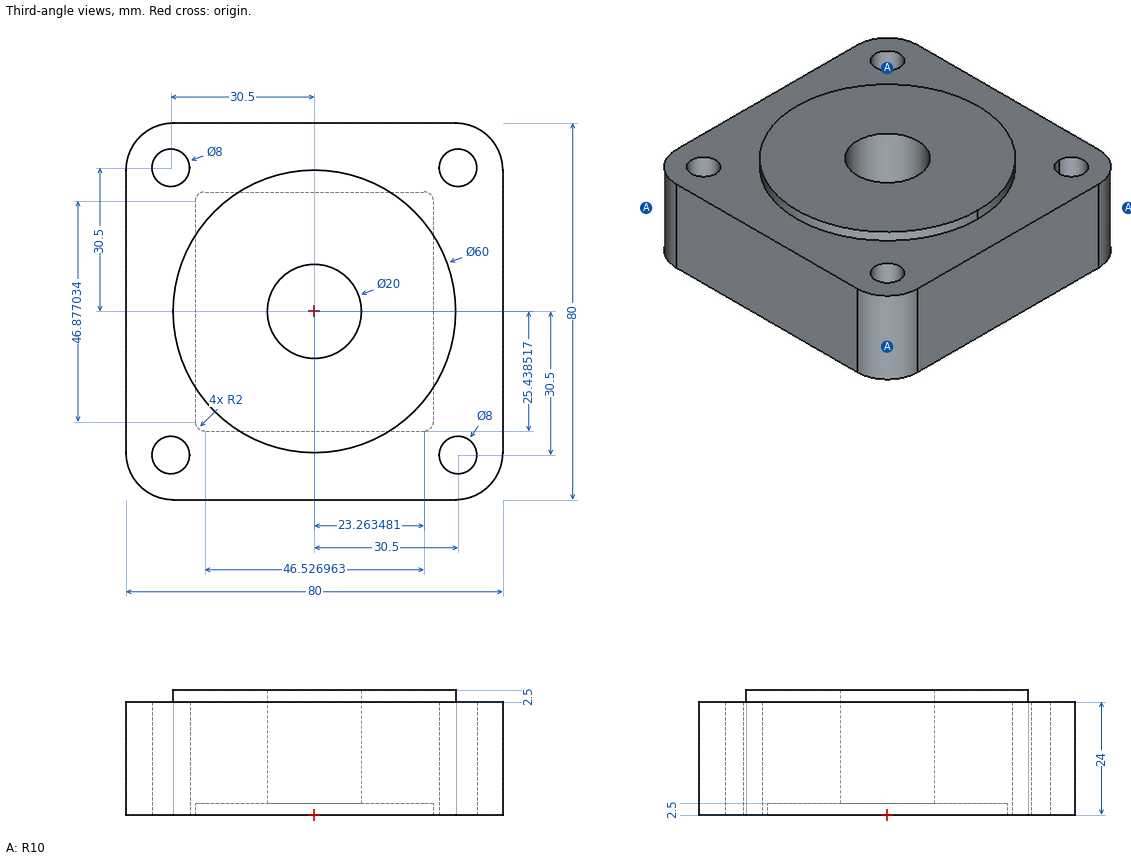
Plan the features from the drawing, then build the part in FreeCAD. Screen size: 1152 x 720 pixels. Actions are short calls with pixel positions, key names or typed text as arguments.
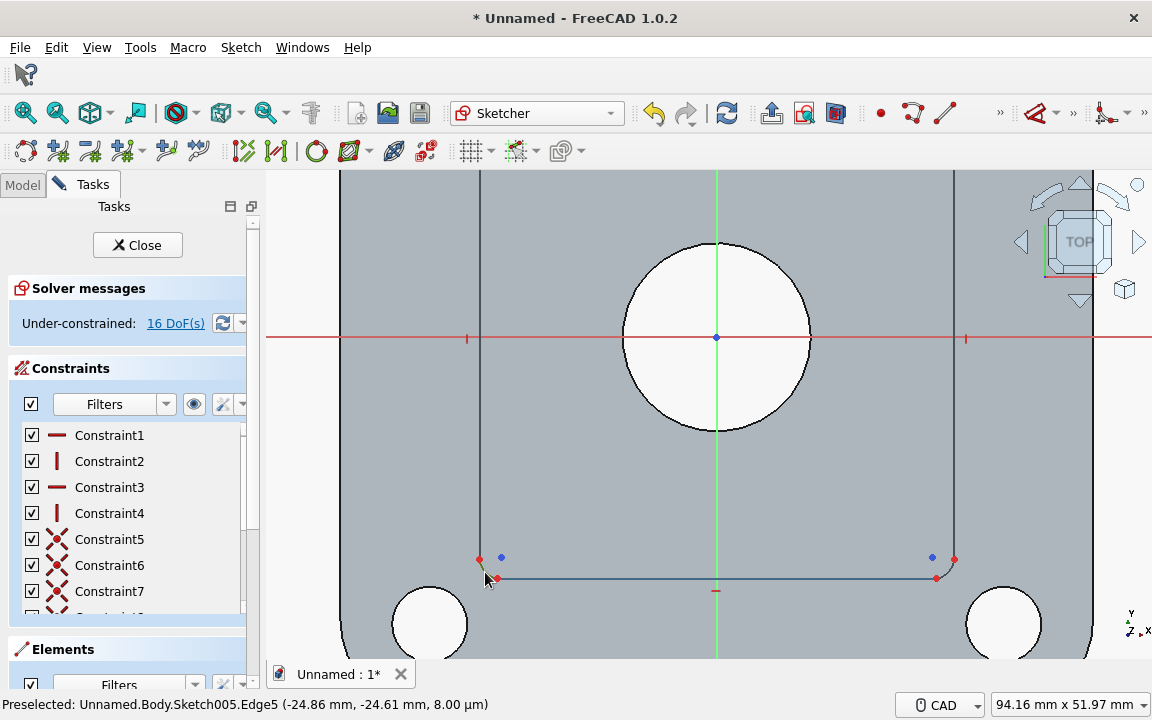
key(t)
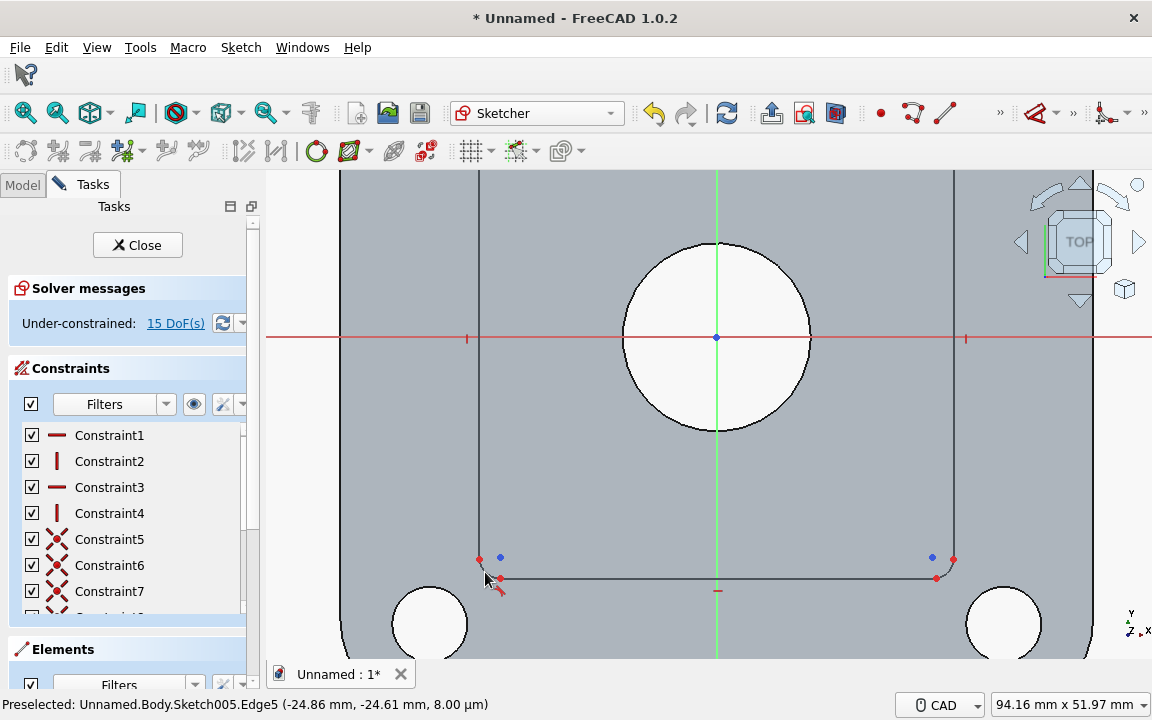
click(805, 579)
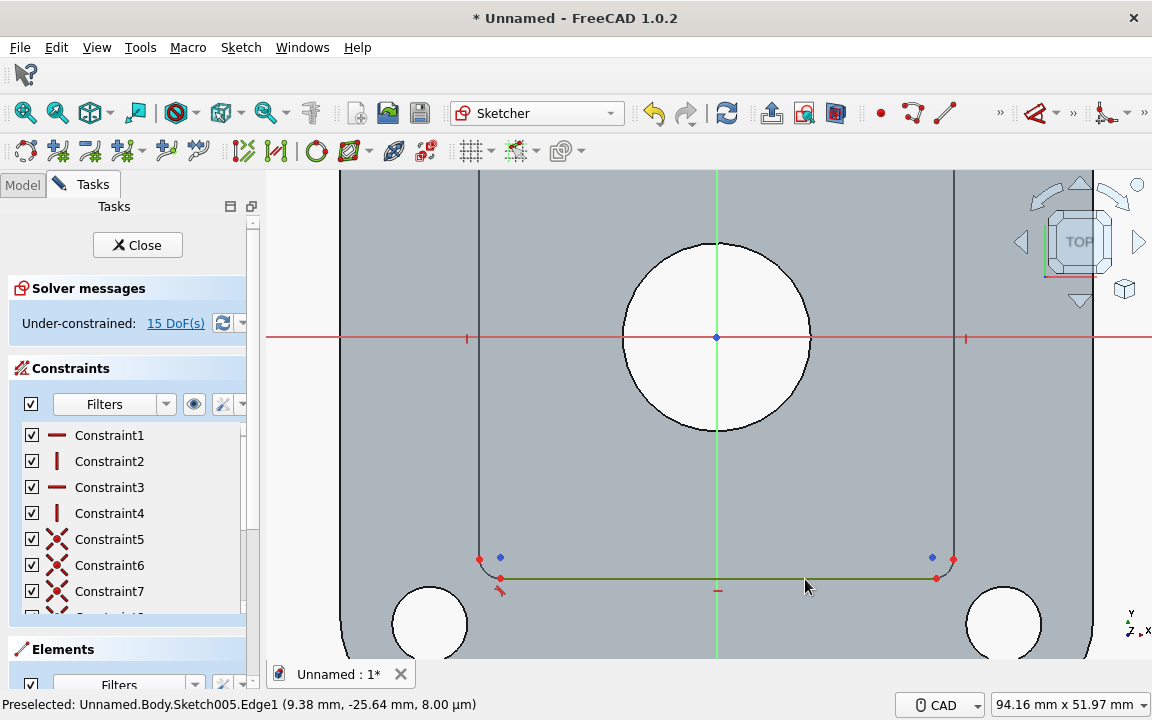
click(948, 572)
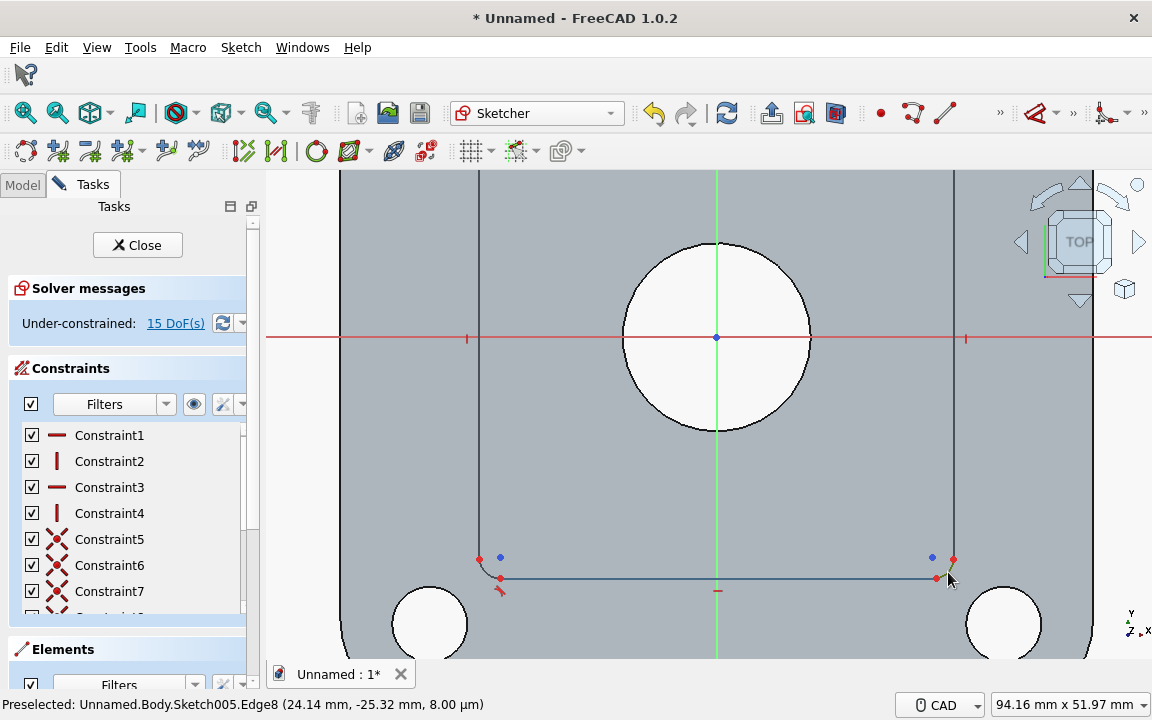
key(t)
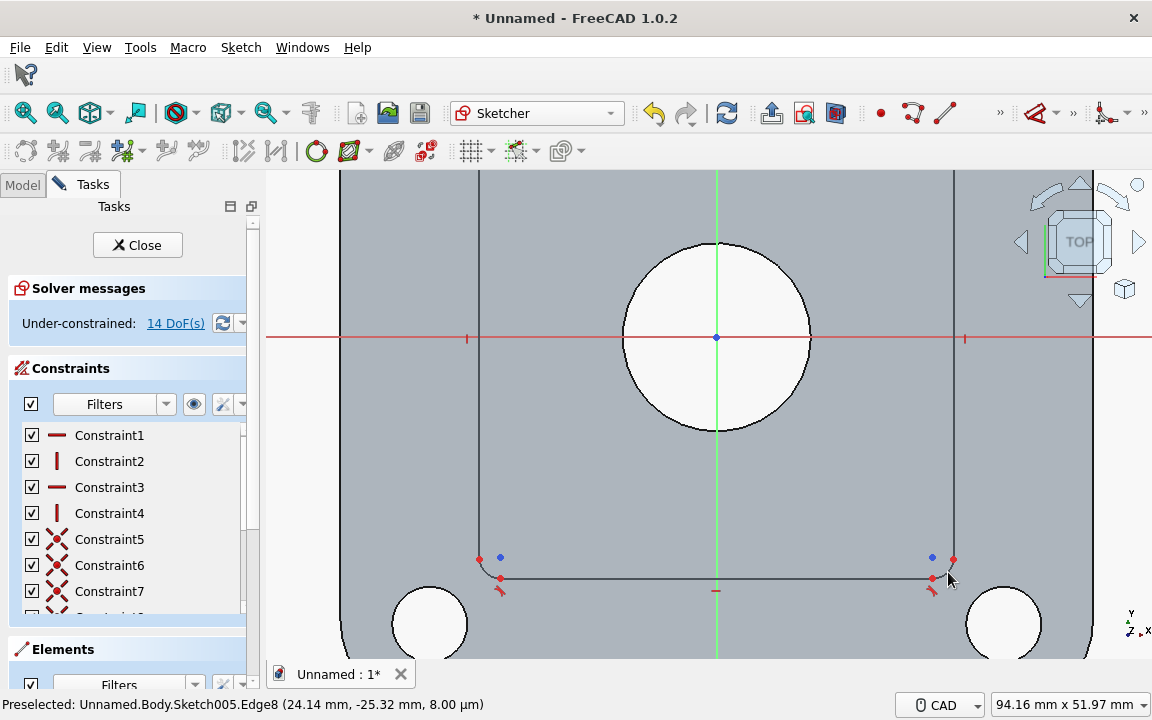
click(479, 427)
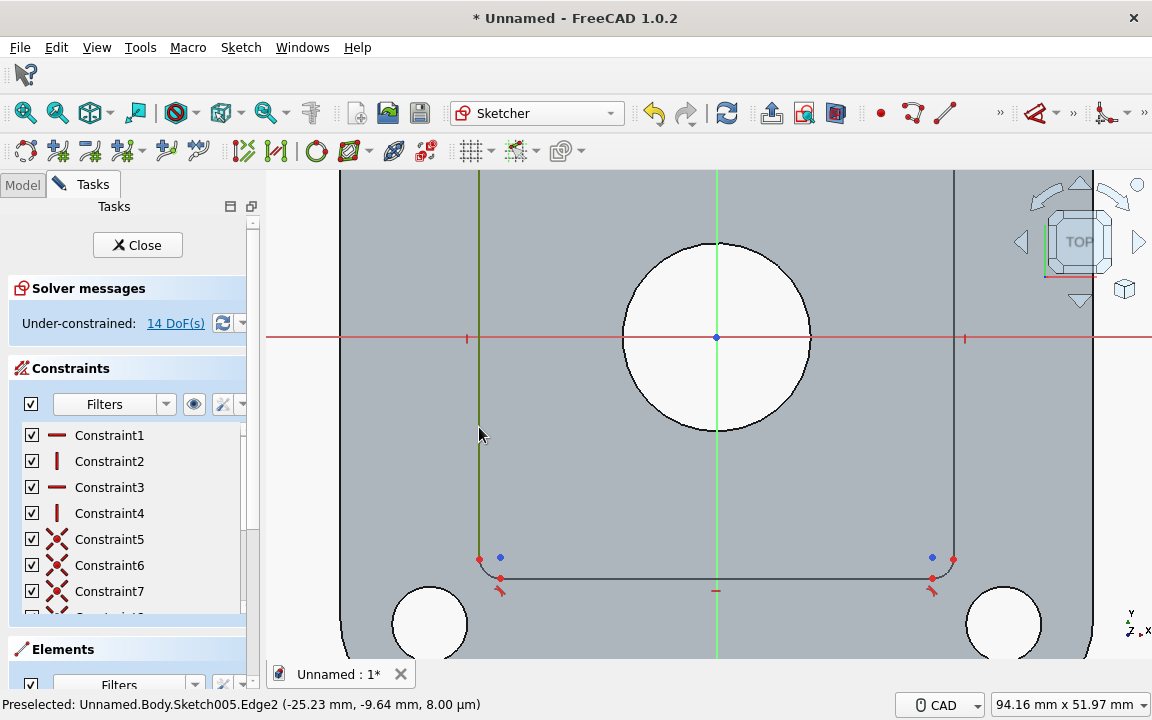
scroll(482, 568, up, 2)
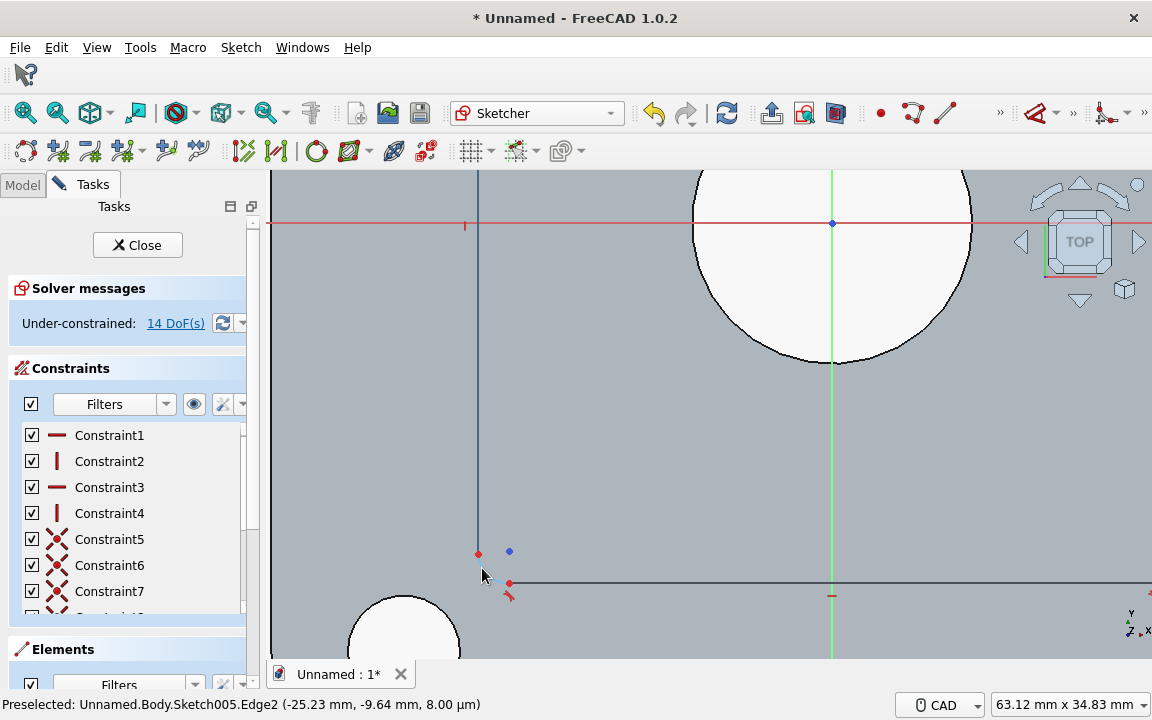
click(482, 568)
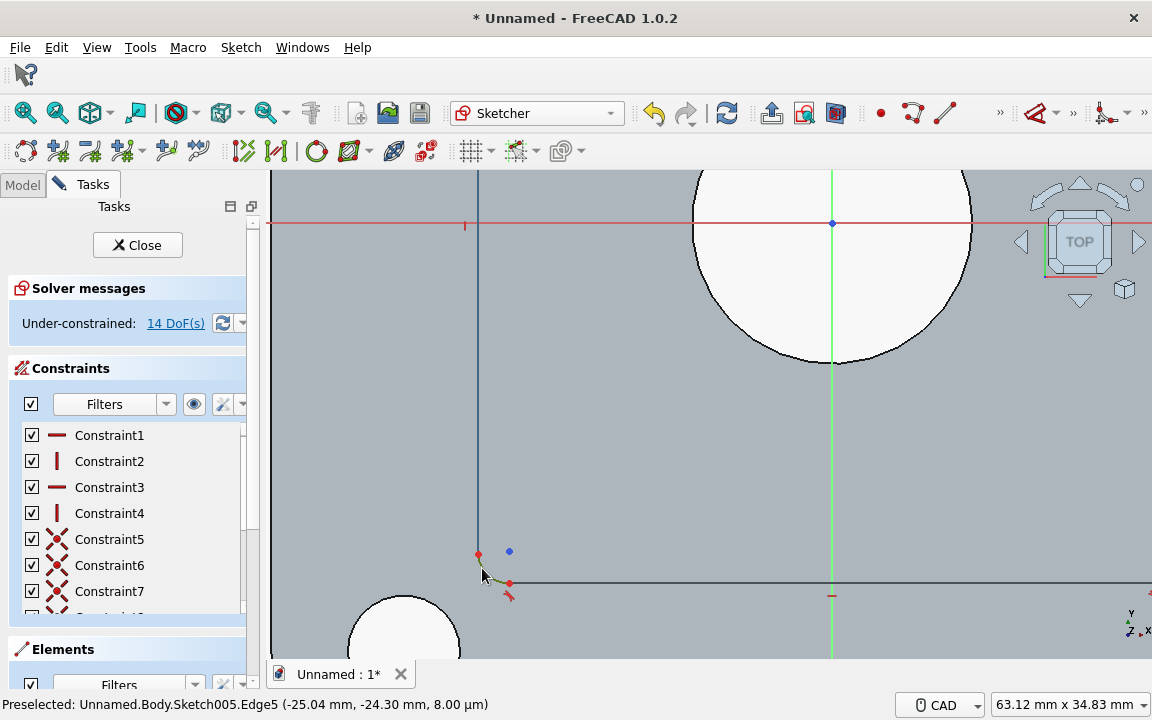
key(t)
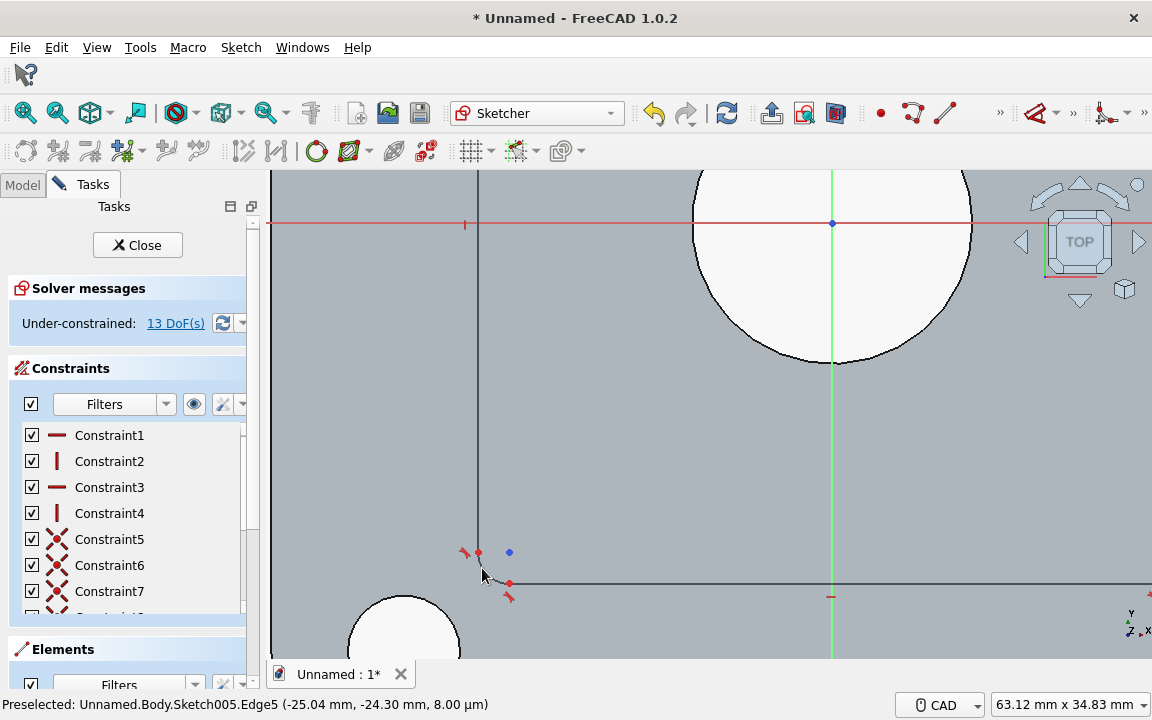
click(478, 355)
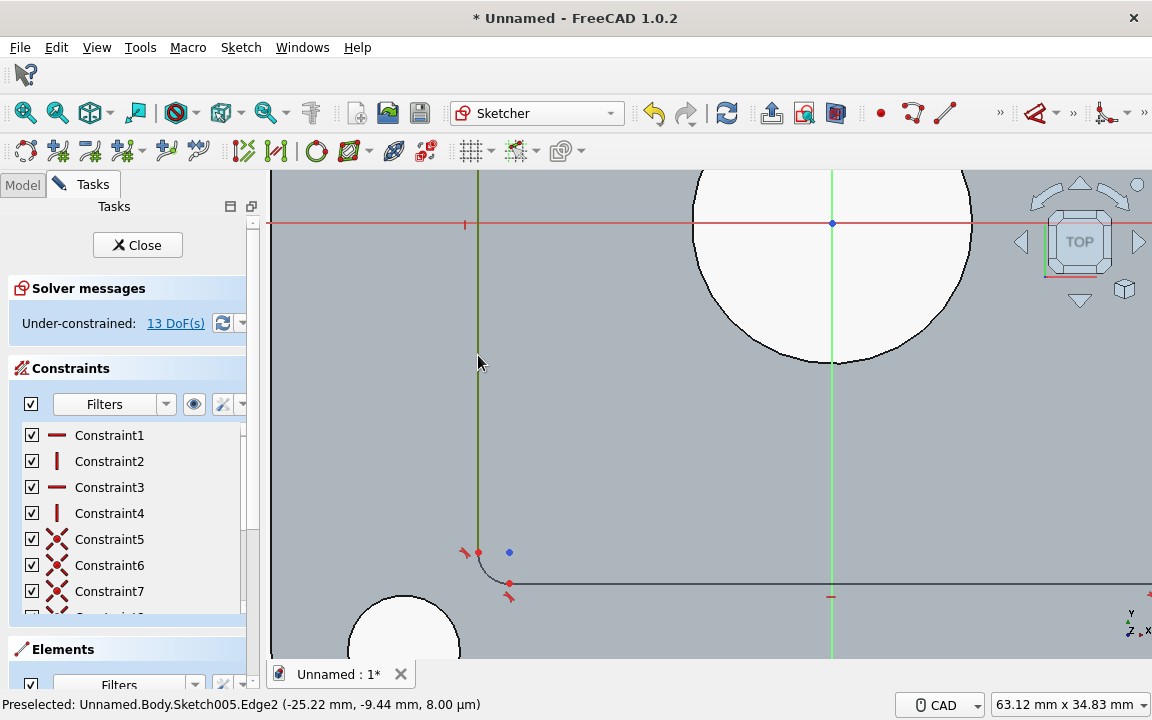
scroll(484, 570, down, 4)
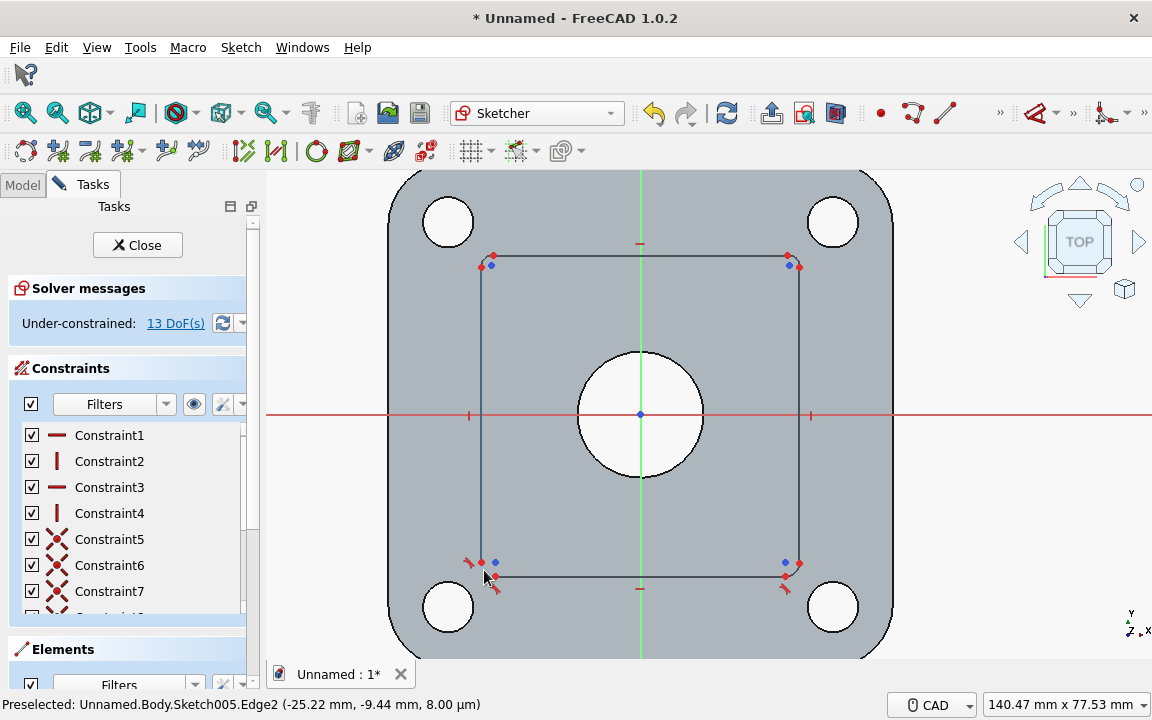
scroll(488, 256, up, 5)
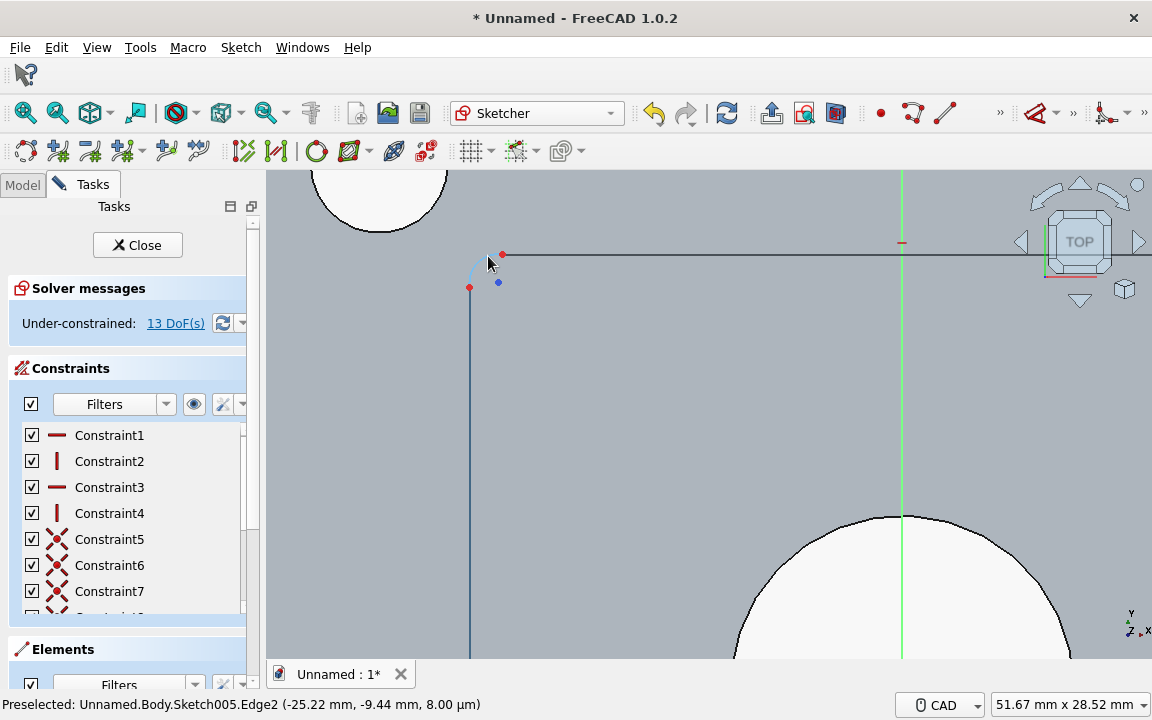
click(487, 256)